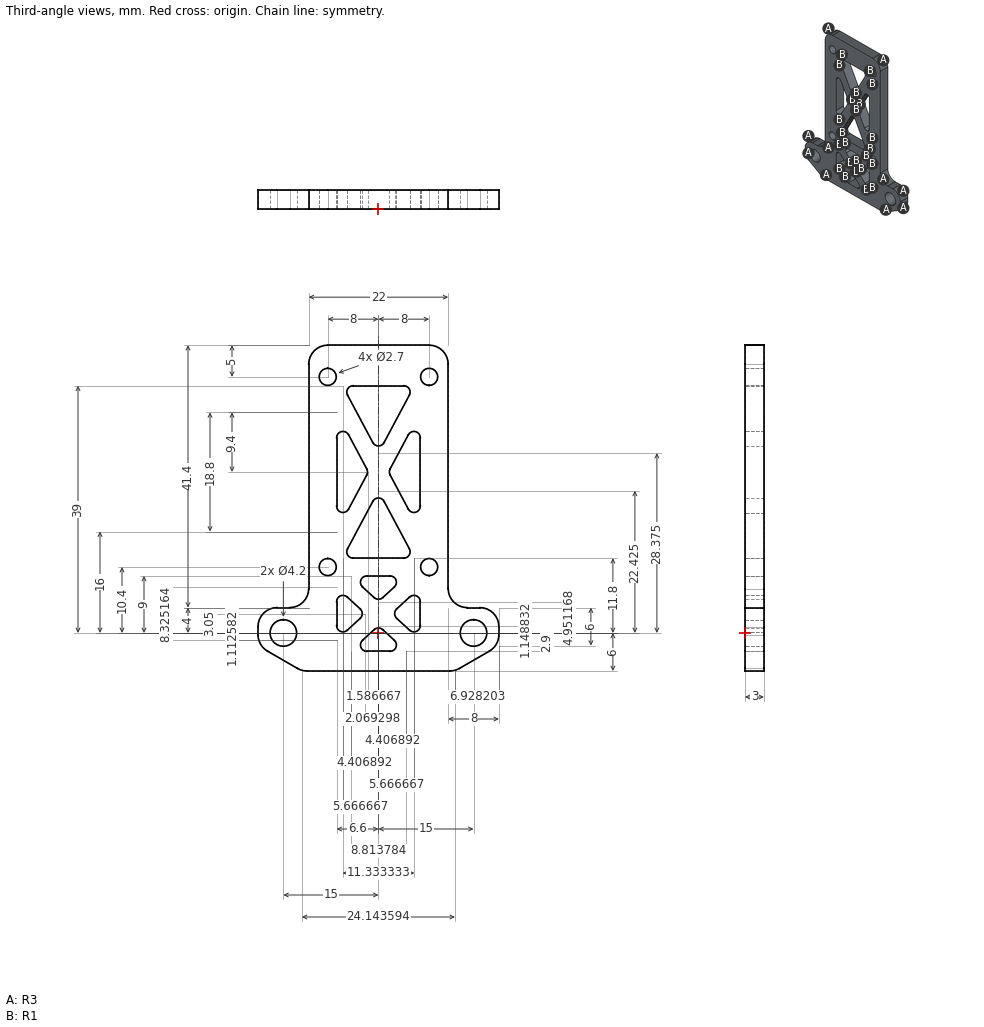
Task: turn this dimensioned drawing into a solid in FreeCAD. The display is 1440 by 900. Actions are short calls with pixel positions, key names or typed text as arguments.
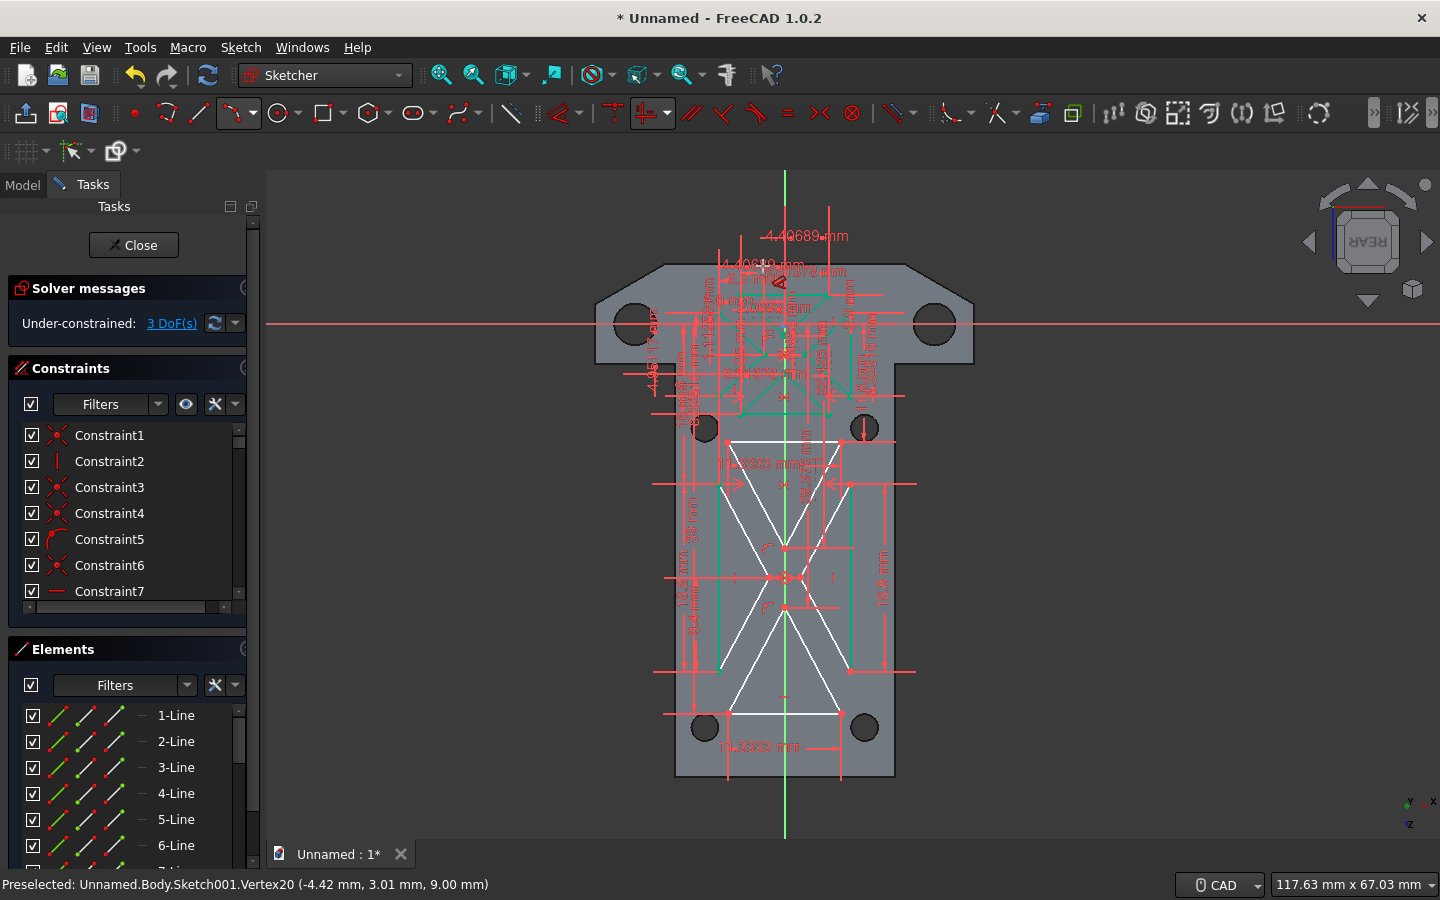
click(841, 442)
click(826, 500)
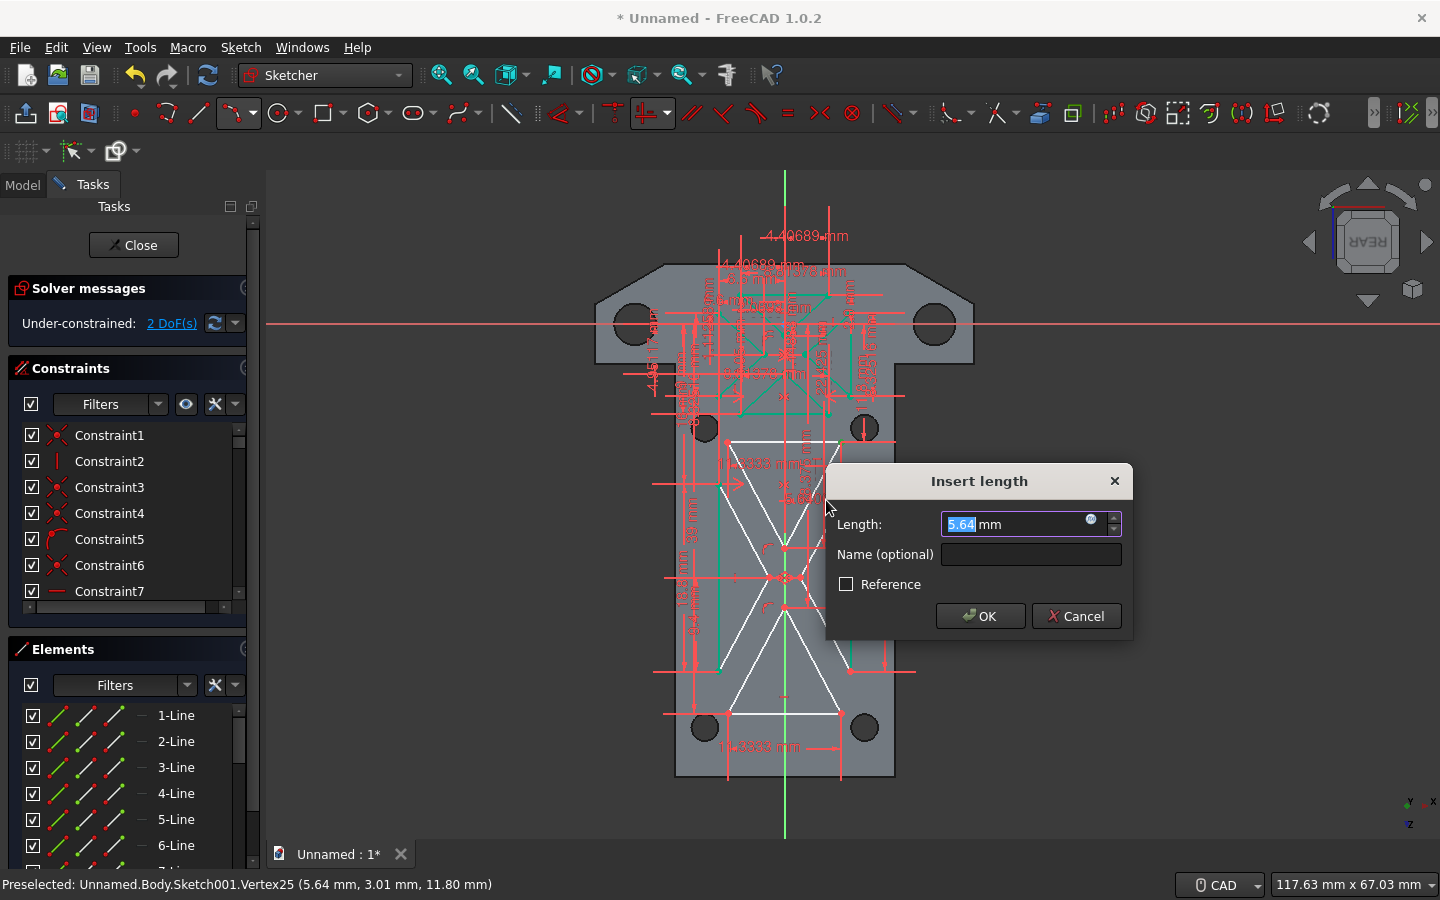
text(5.666667)
key(Return)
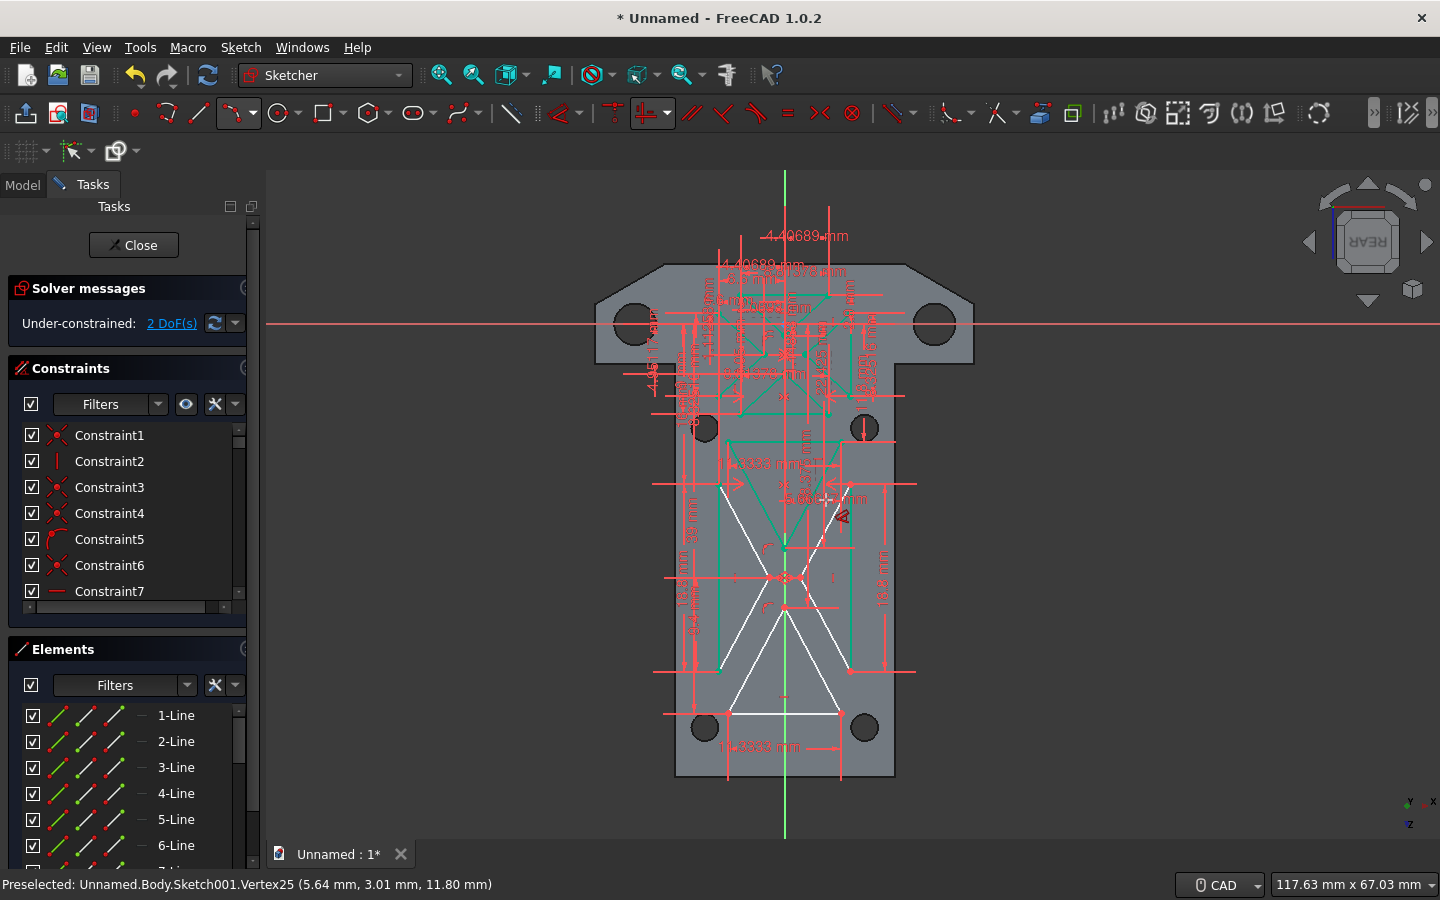
scroll(769, 578, up, 5)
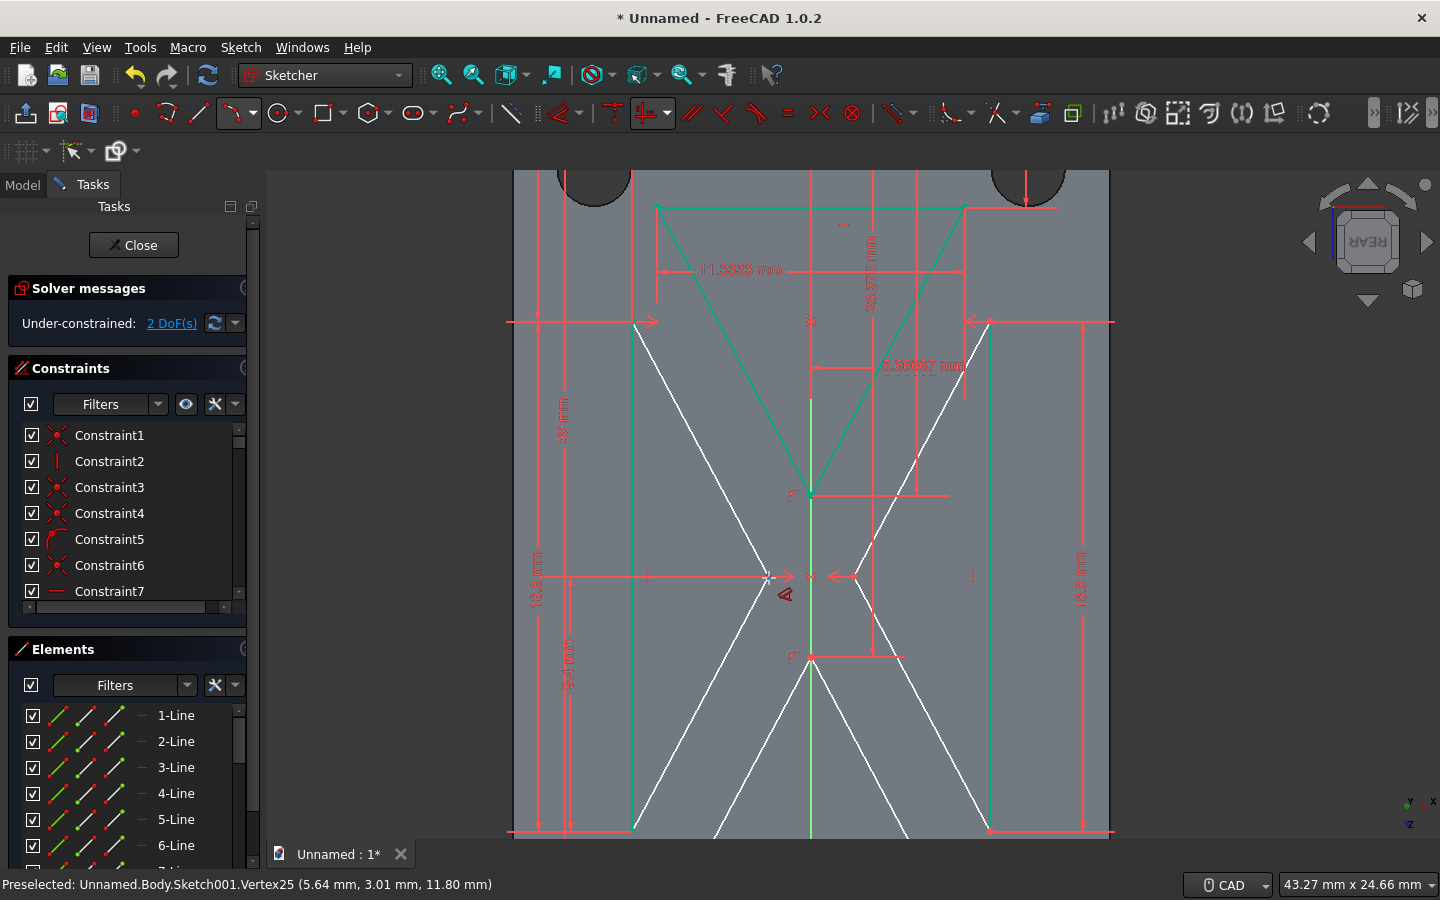
click(769, 577)
click(790, 611)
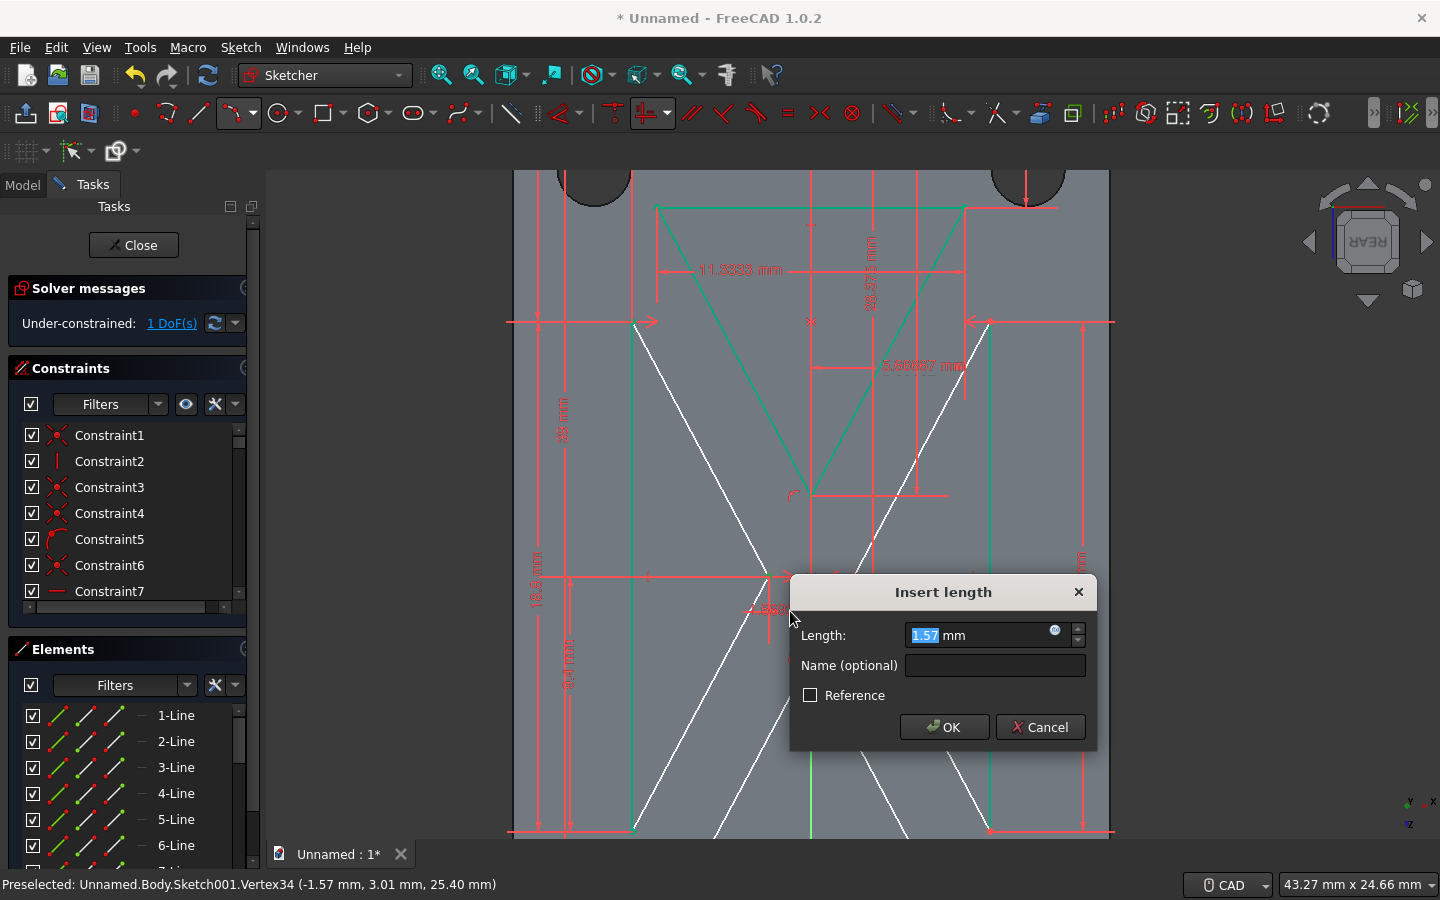
text(1.586667)
key(Return)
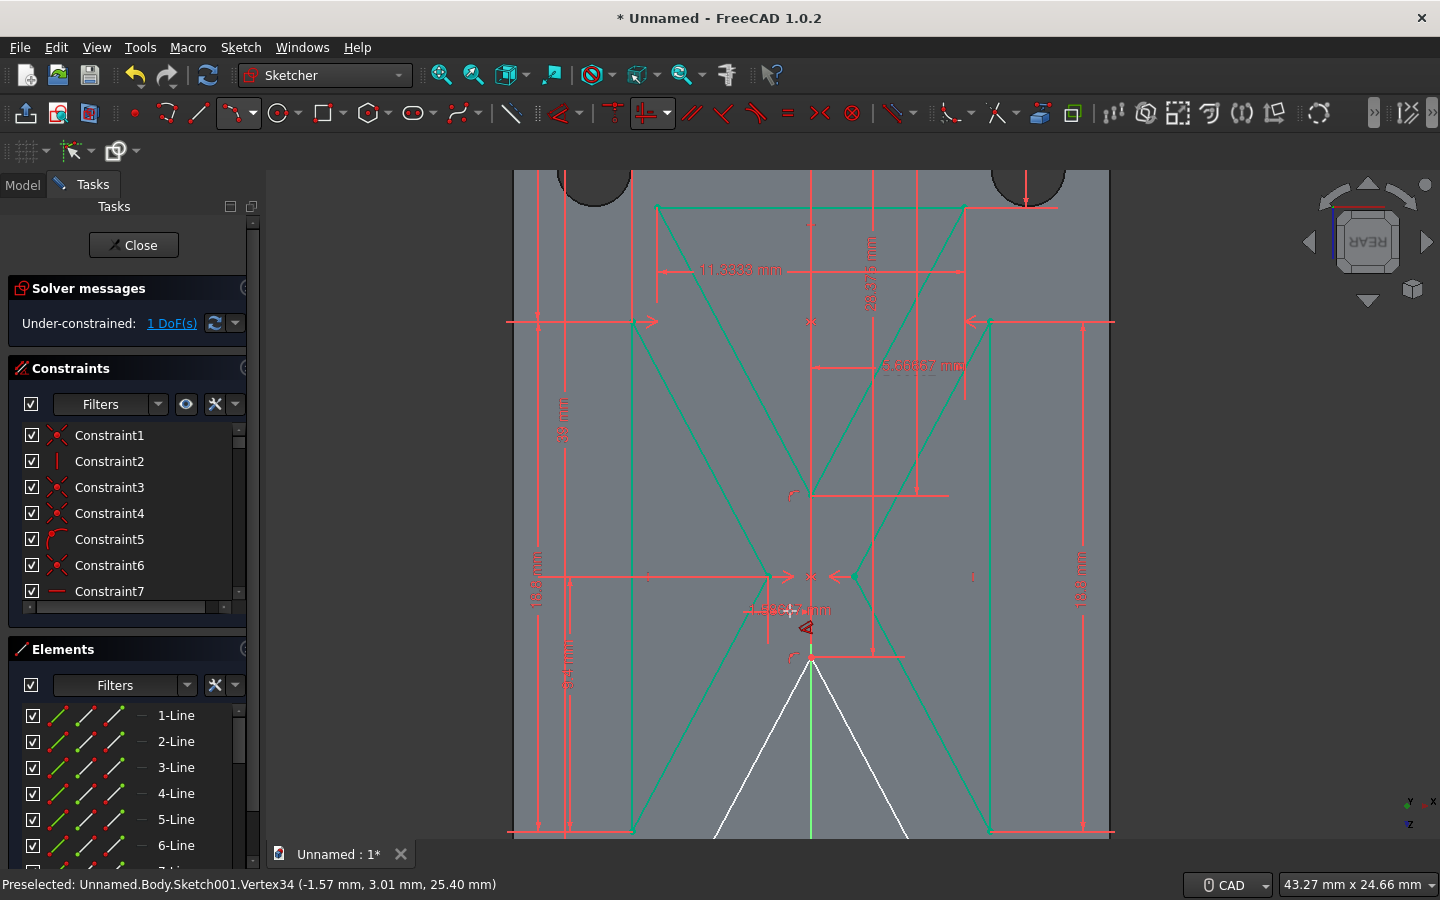
scroll(769, 579, down, 5)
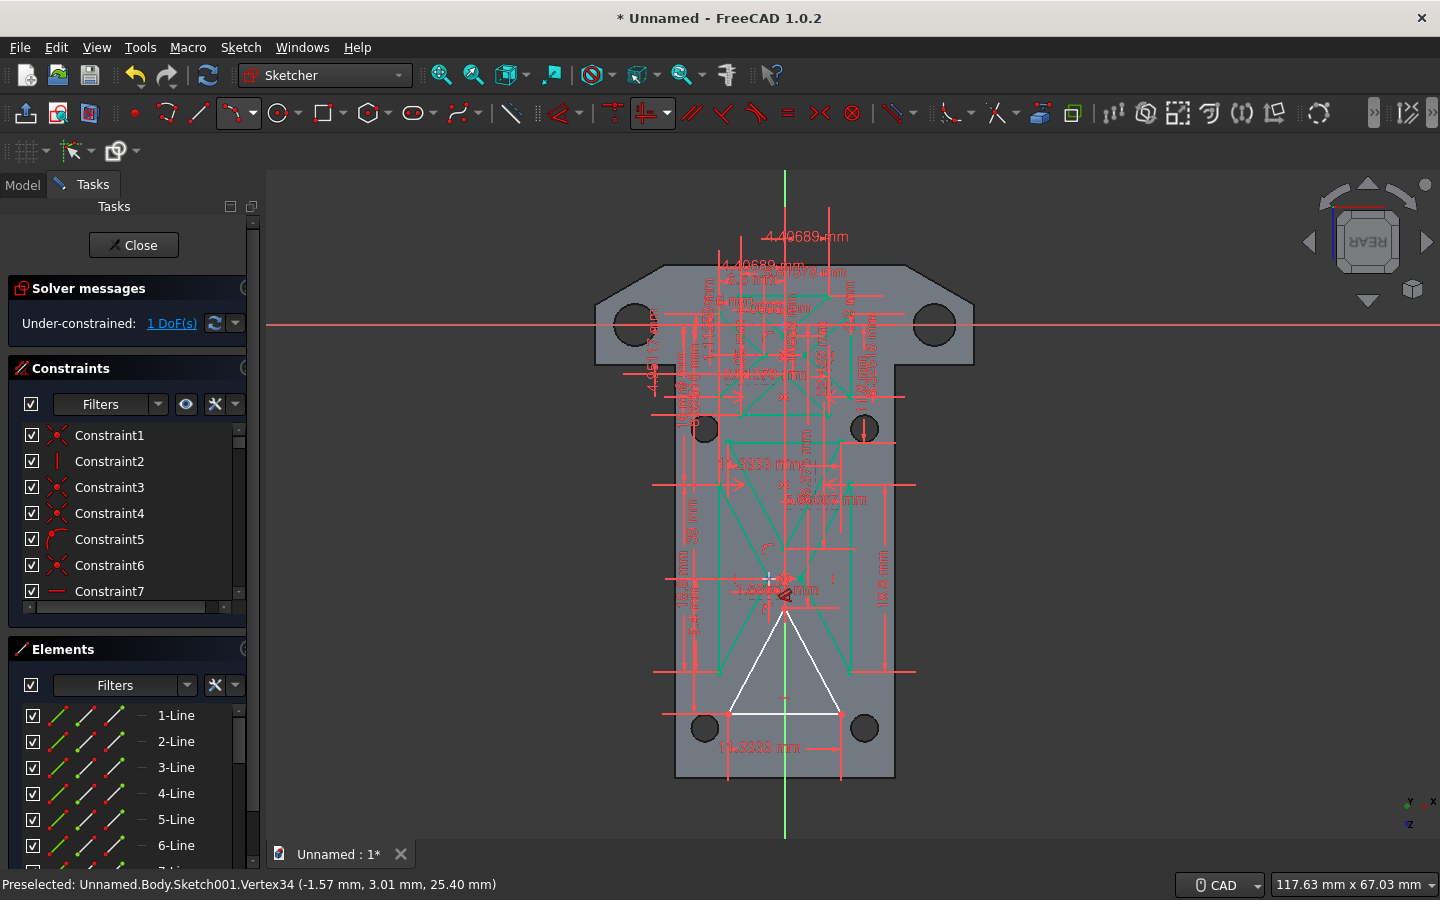
click(728, 714)
click(756, 772)